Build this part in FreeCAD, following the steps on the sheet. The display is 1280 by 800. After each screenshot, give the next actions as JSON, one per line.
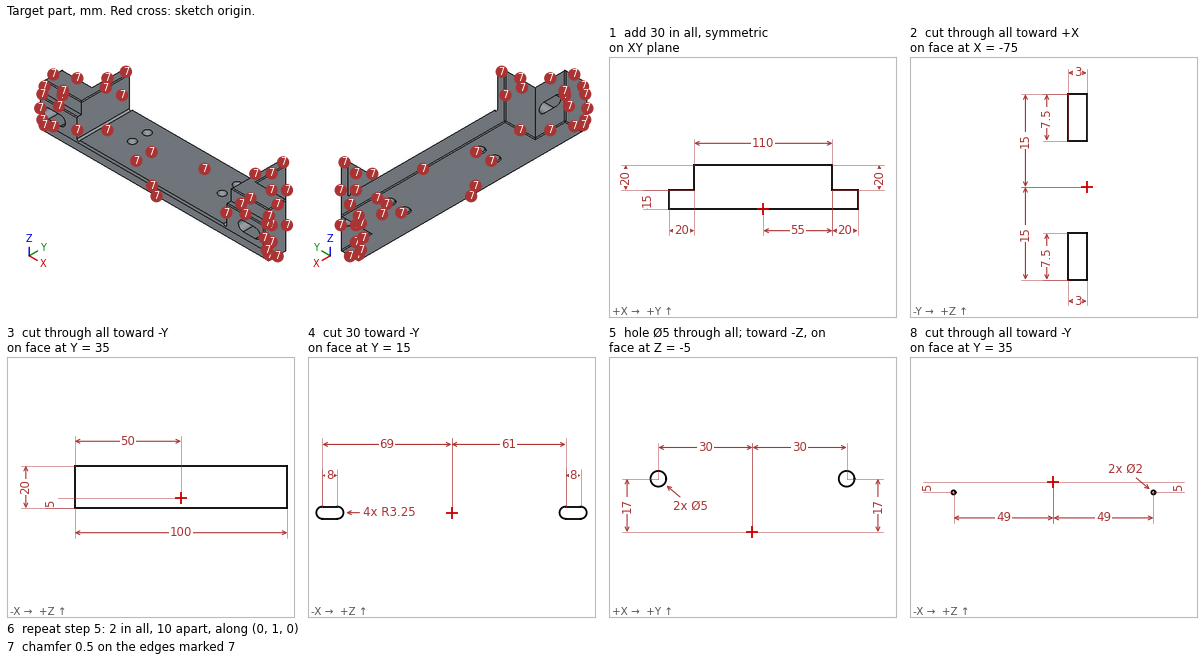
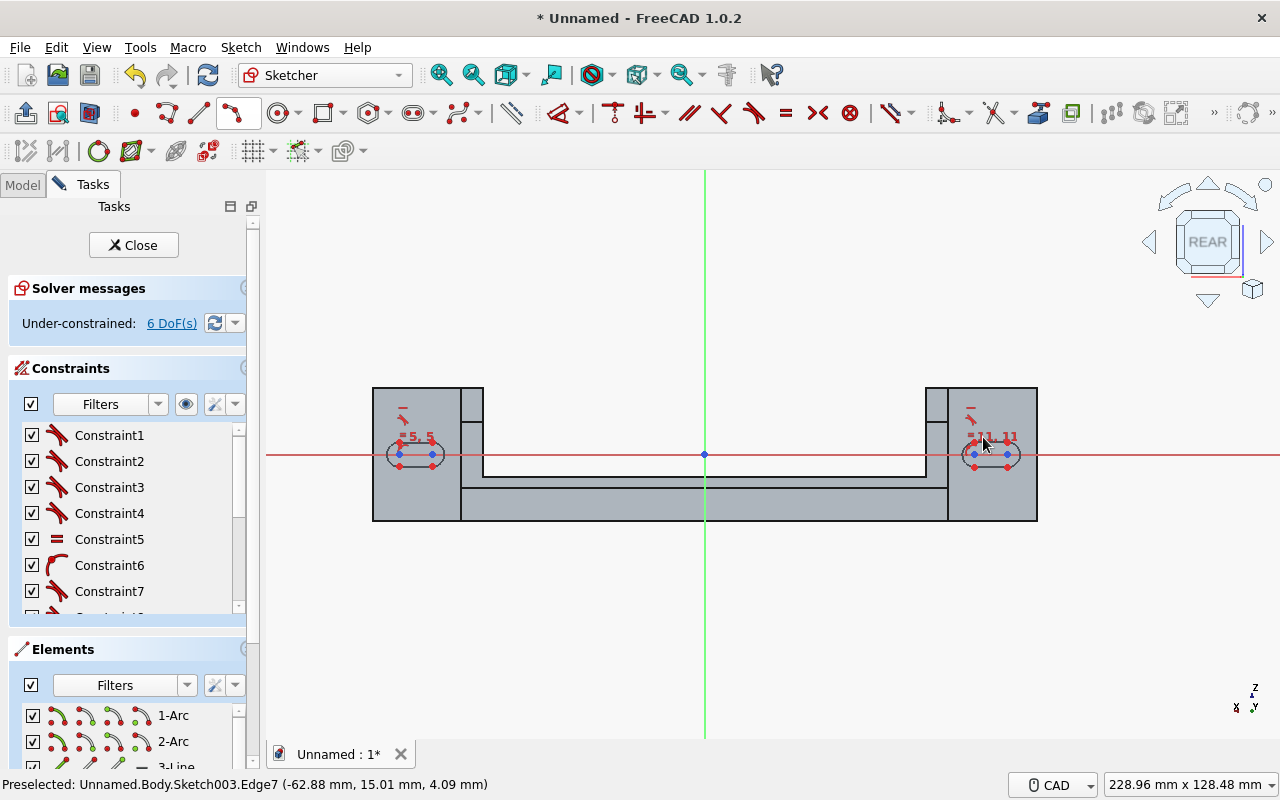
{"action": "scroll", "coordinate": [389, 448], "scroll_direction": "up", "scroll_amount": 4}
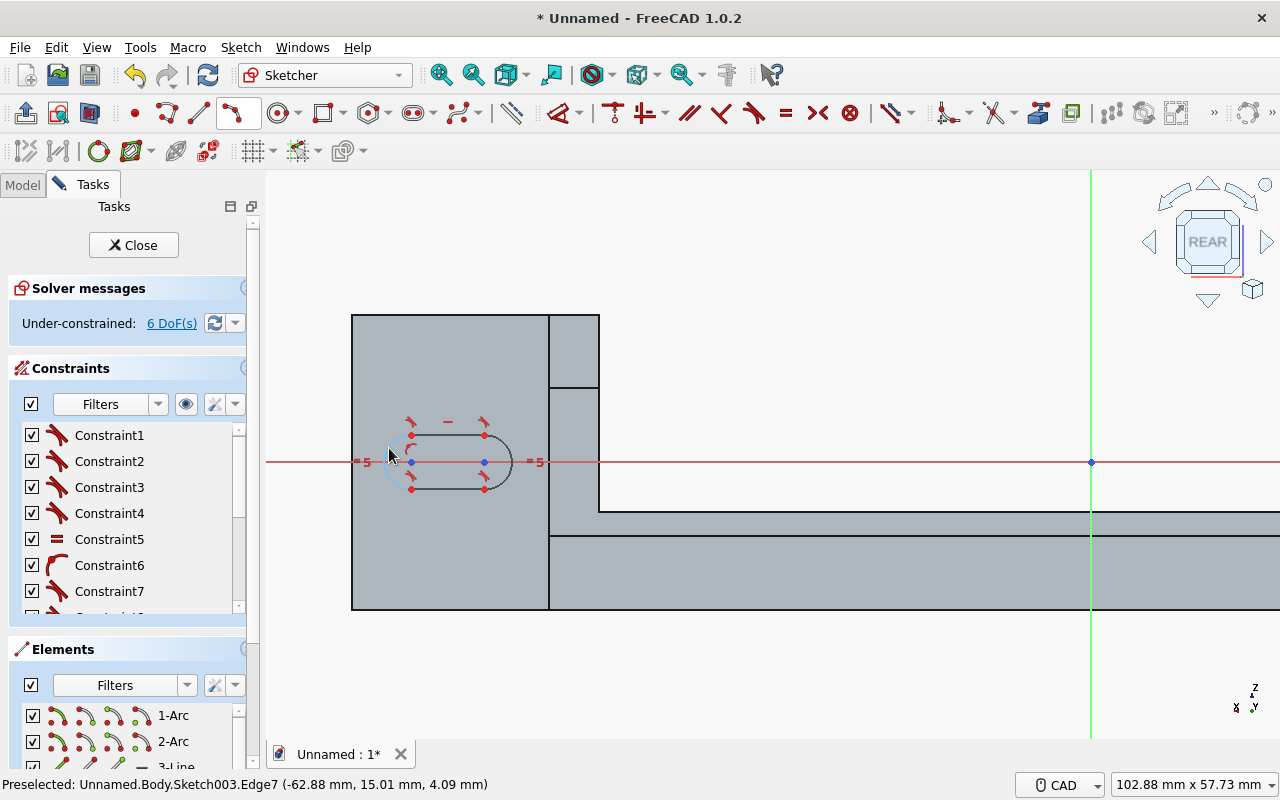
{"action": "left_click", "coordinate": [389, 446]}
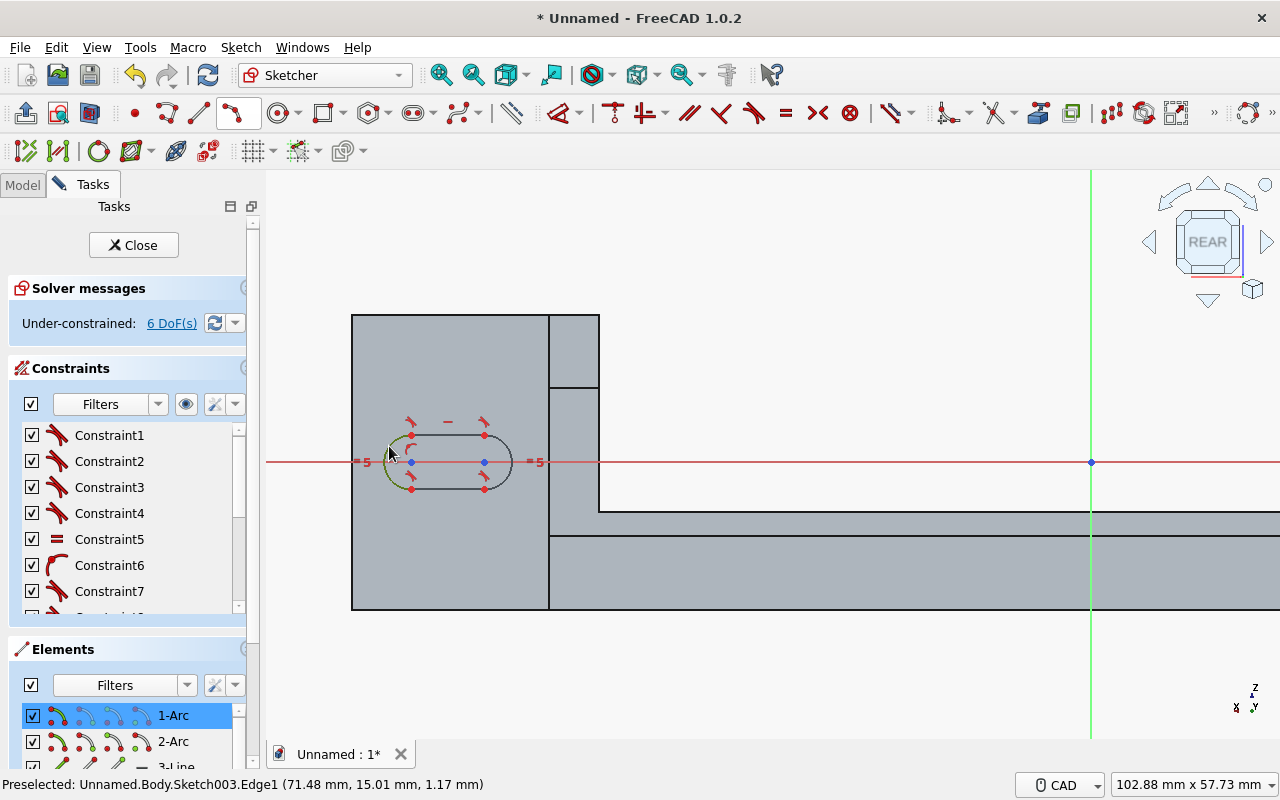
{"action": "scroll", "coordinate": [389, 448], "scroll_direction": "down", "scroll_amount": 4}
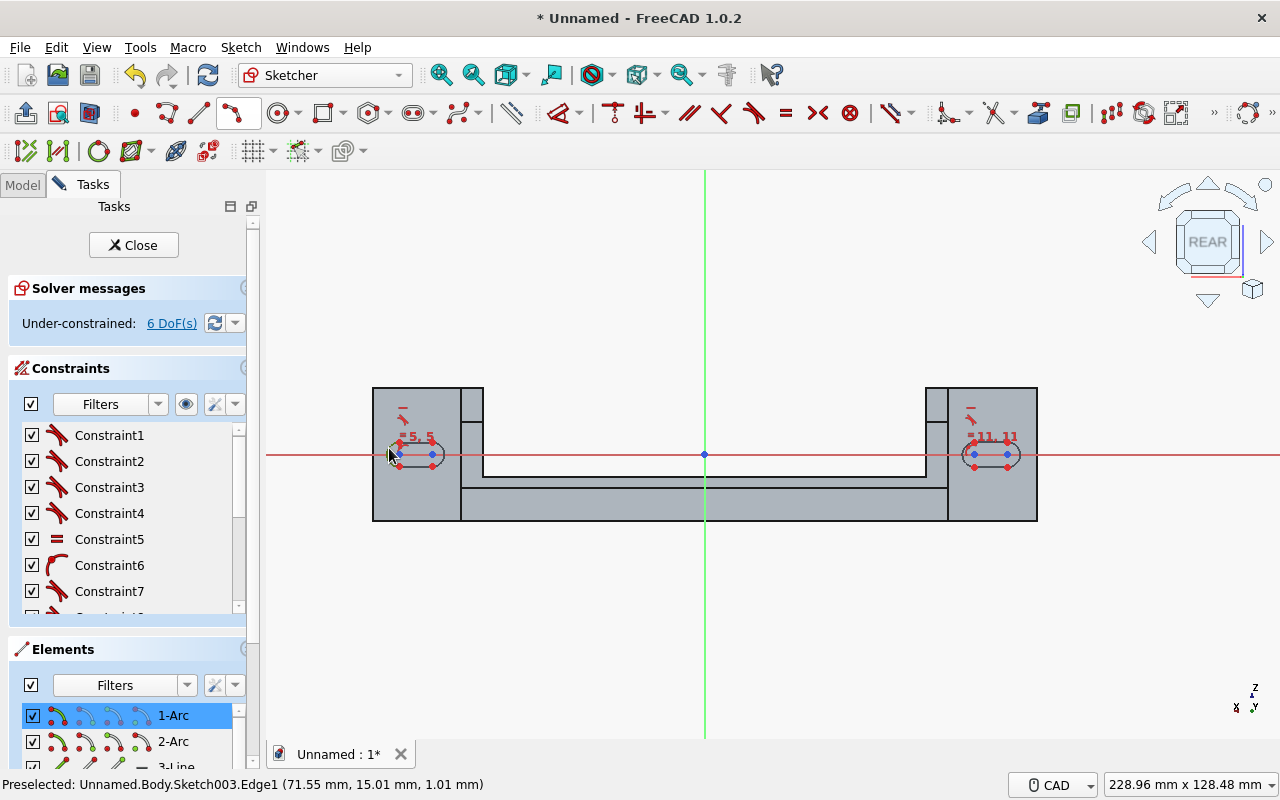
{"action": "scroll", "coordinate": [965, 447], "scroll_direction": "up", "scroll_amount": 4}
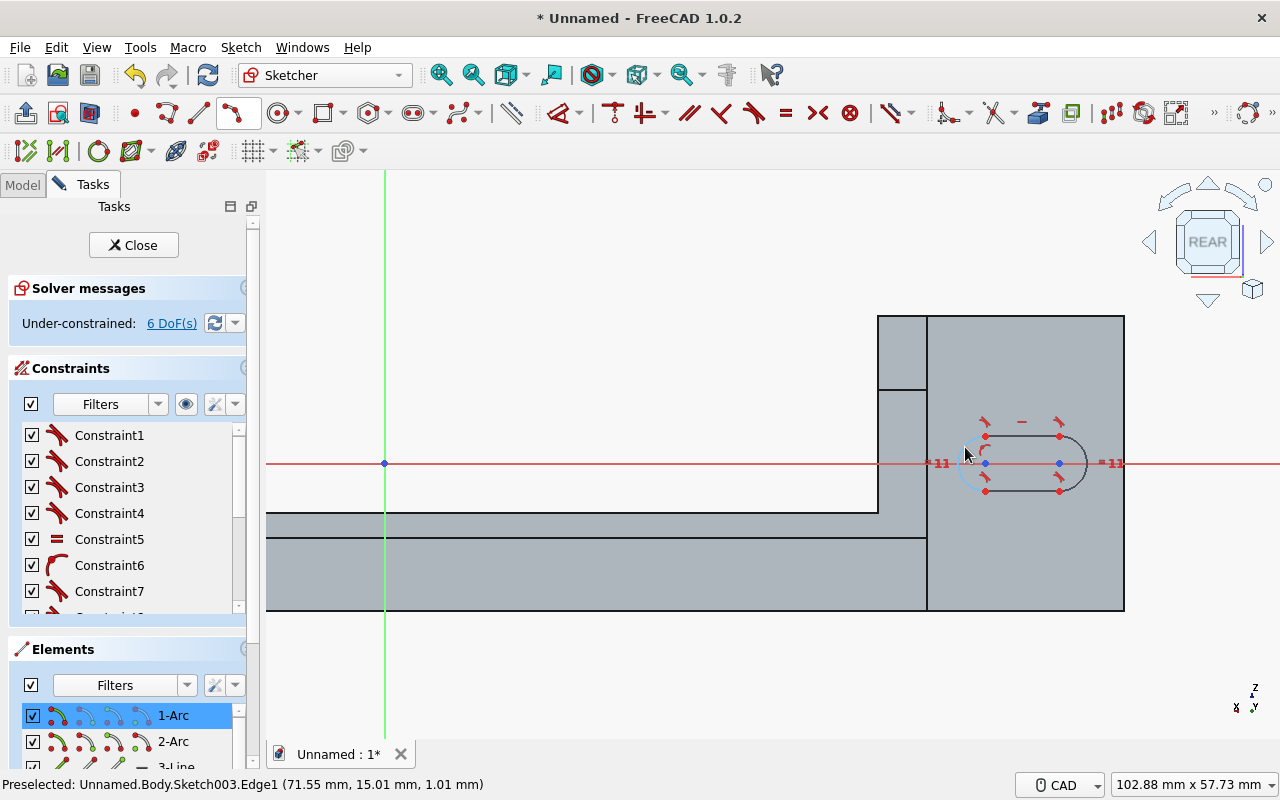
{"action": "left_click", "coordinate": [964, 447]}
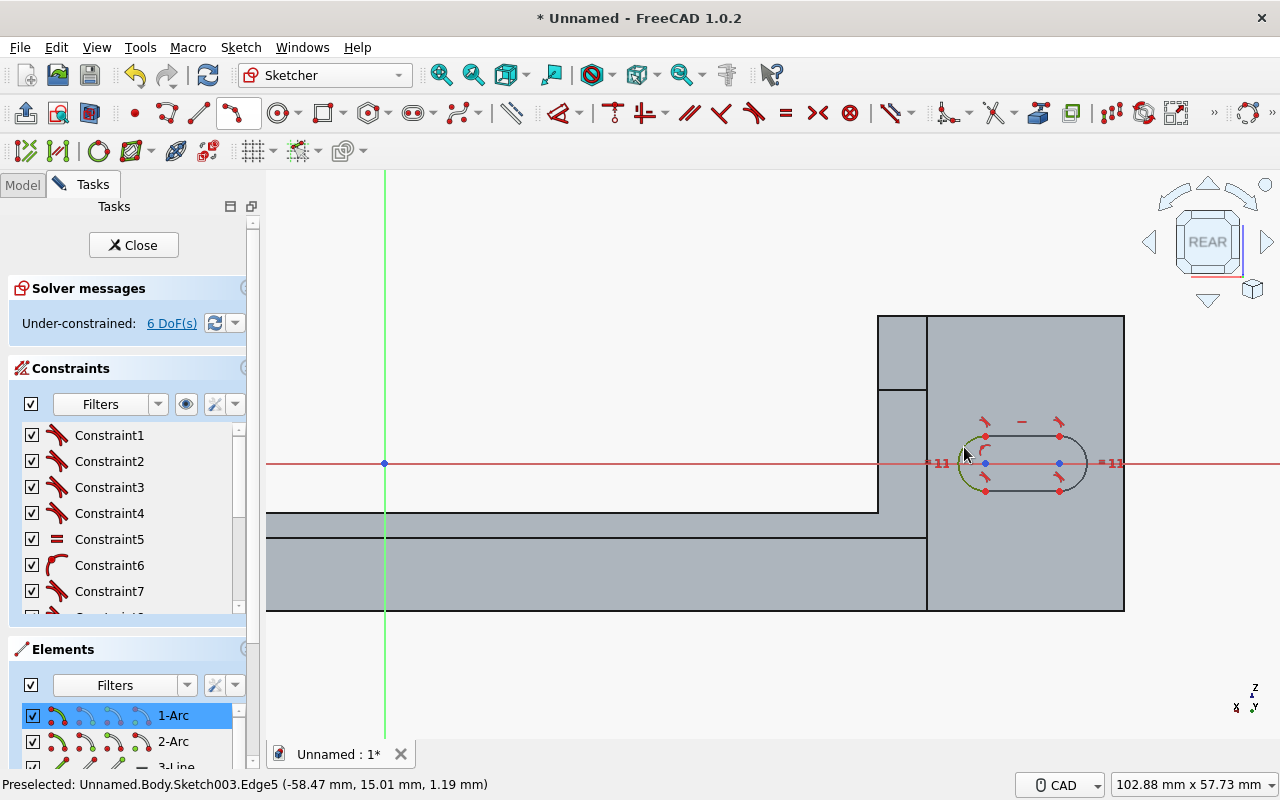
{"action": "key", "text": "e"}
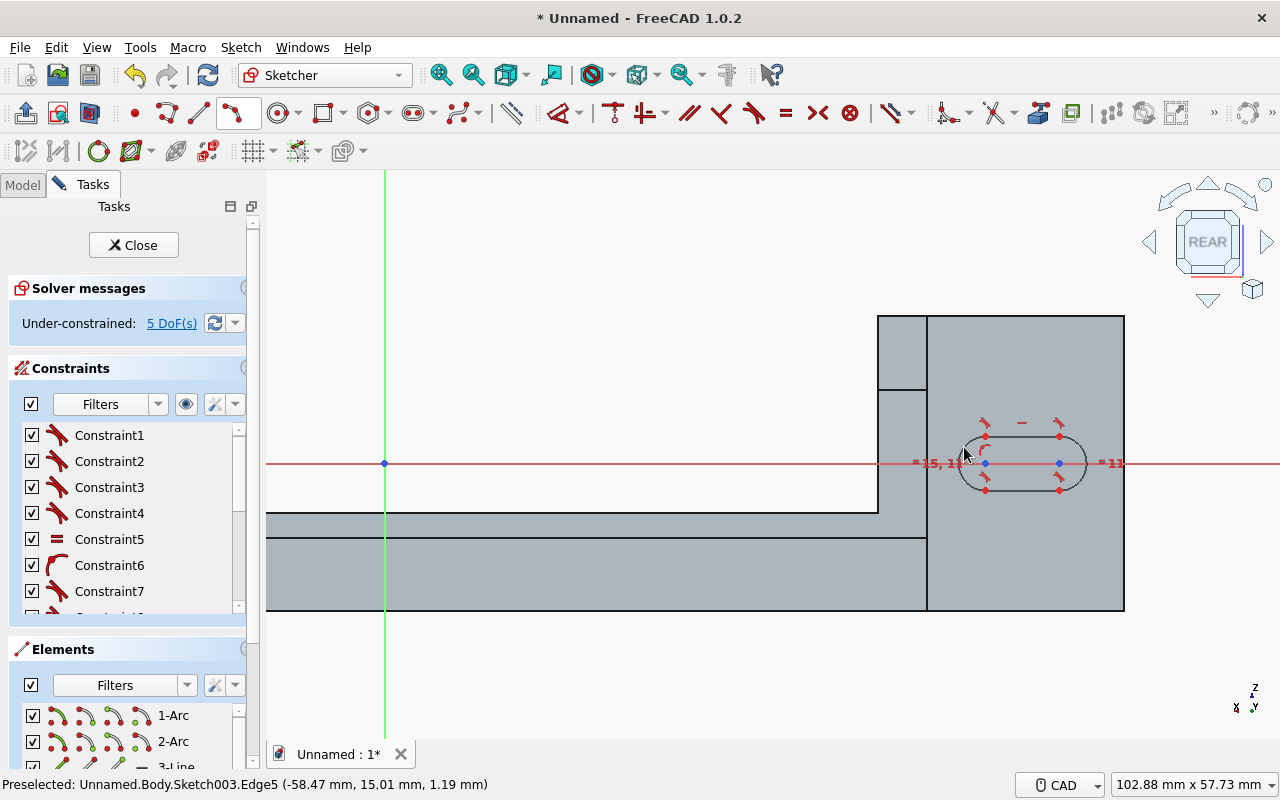
{"action": "key", "text": "d"}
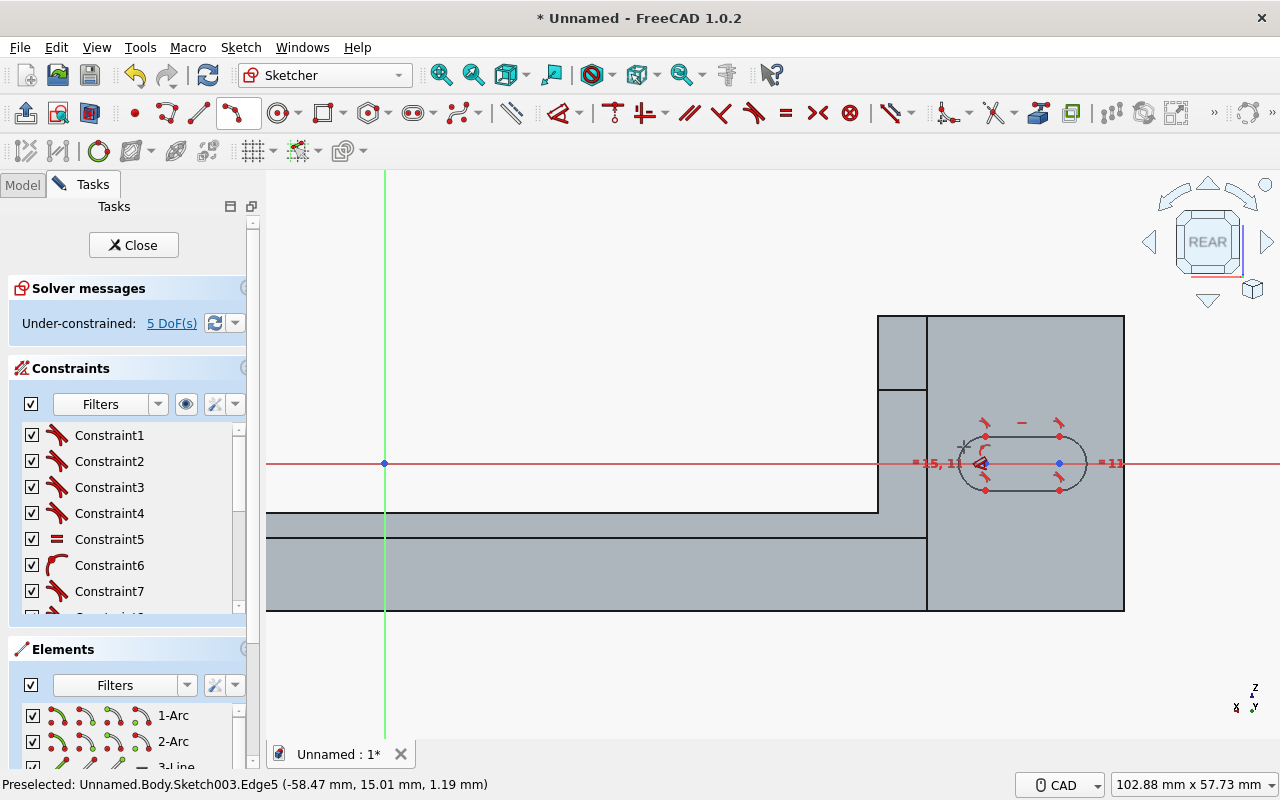
{"action": "scroll", "coordinate": [965, 447], "scroll_direction": "down", "scroll_amount": 4}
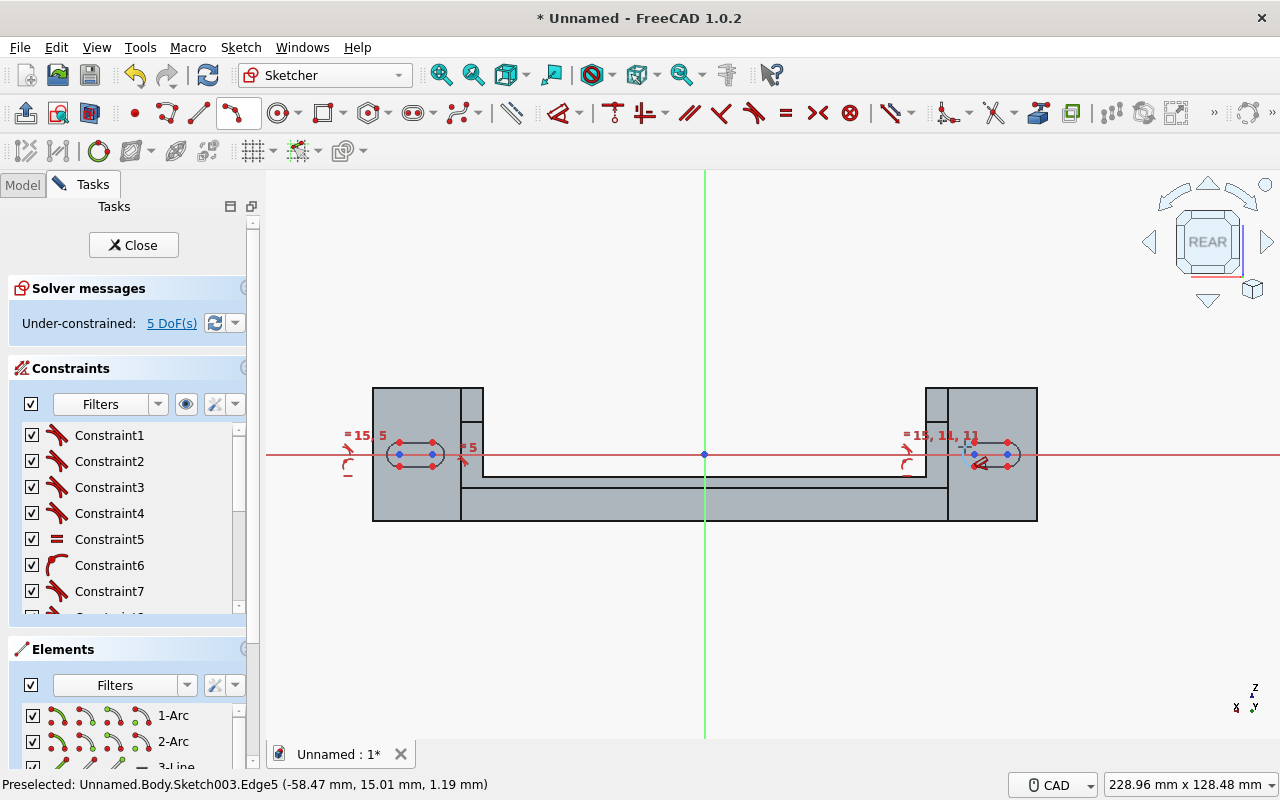
{"action": "scroll", "coordinate": [389, 448], "scroll_direction": "up", "scroll_amount": 6}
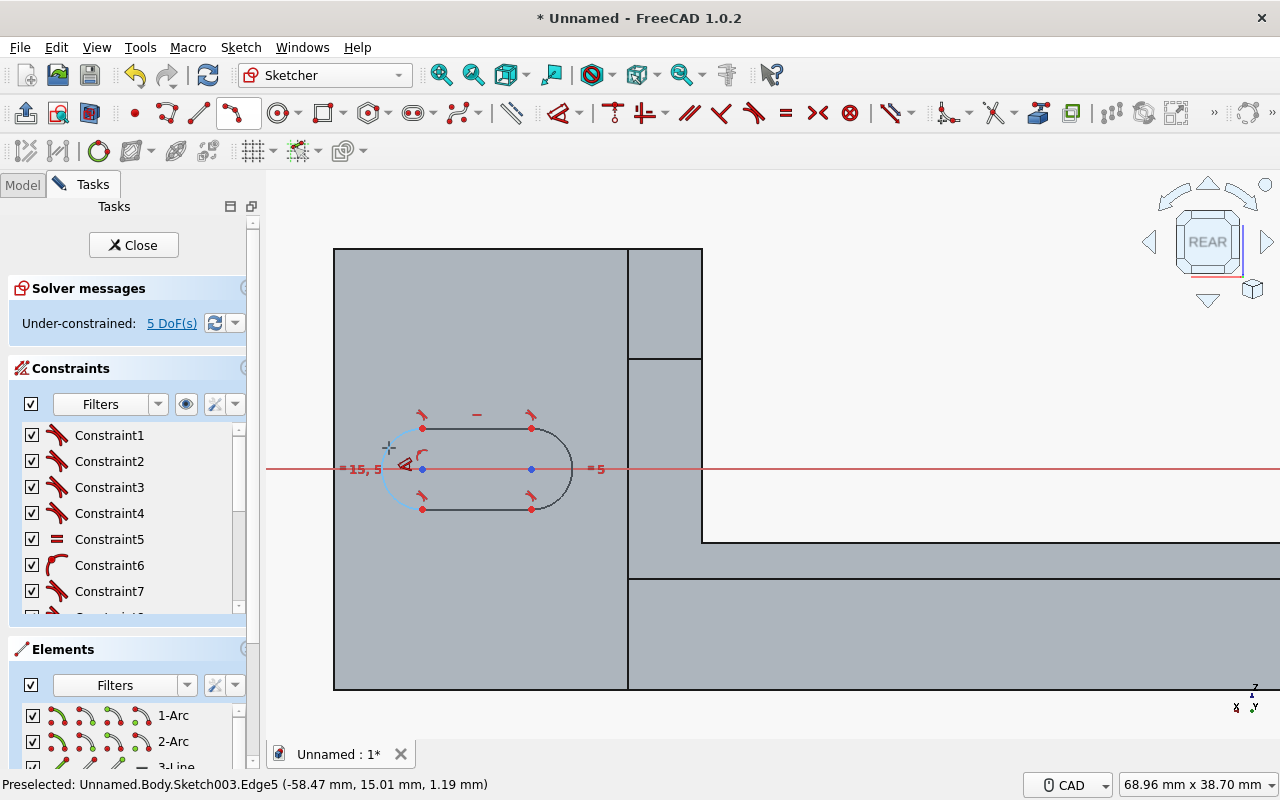
{"action": "left_click", "coordinate": [390, 445]}
{"action": "left_click", "coordinate": [364, 426]}